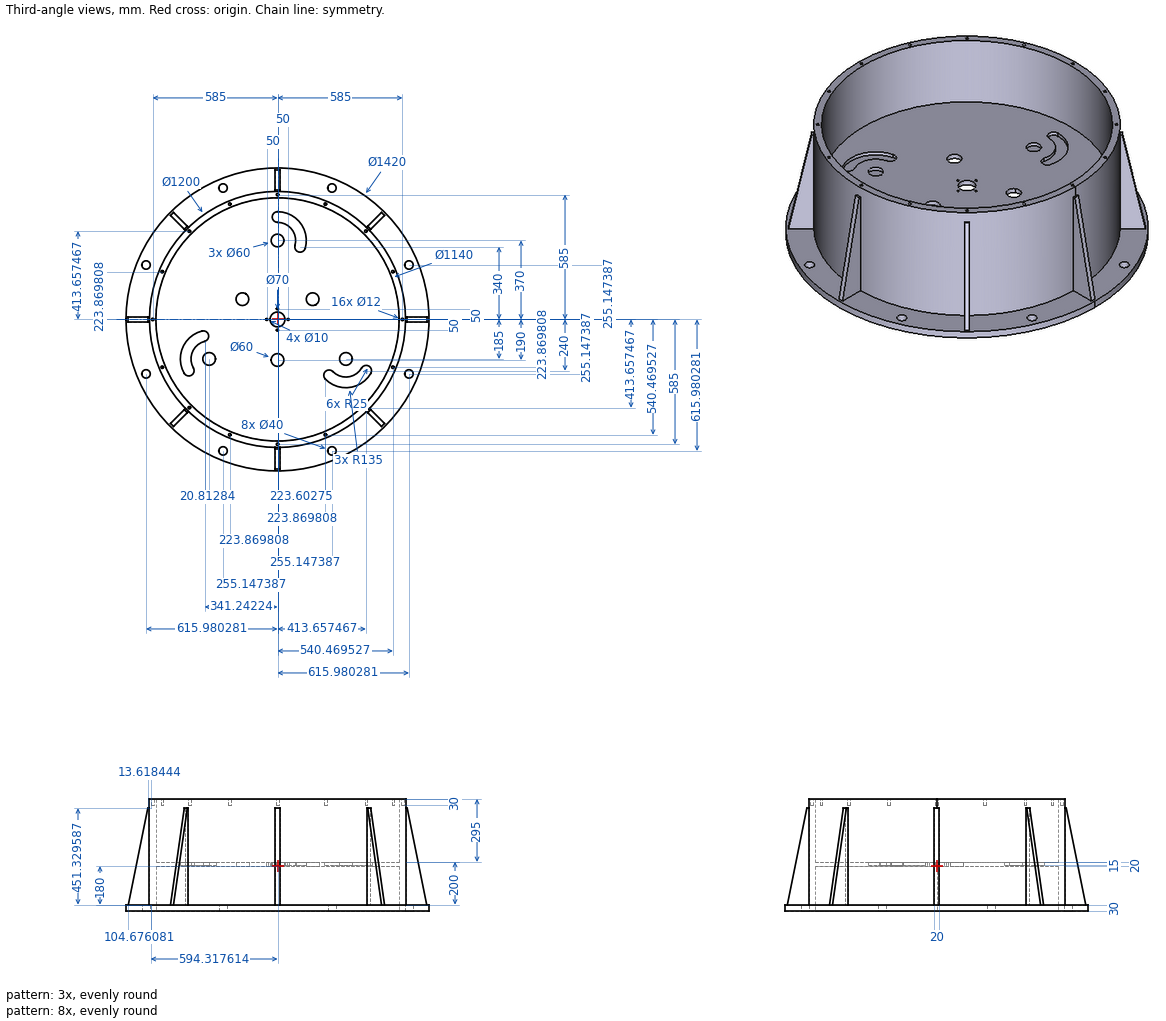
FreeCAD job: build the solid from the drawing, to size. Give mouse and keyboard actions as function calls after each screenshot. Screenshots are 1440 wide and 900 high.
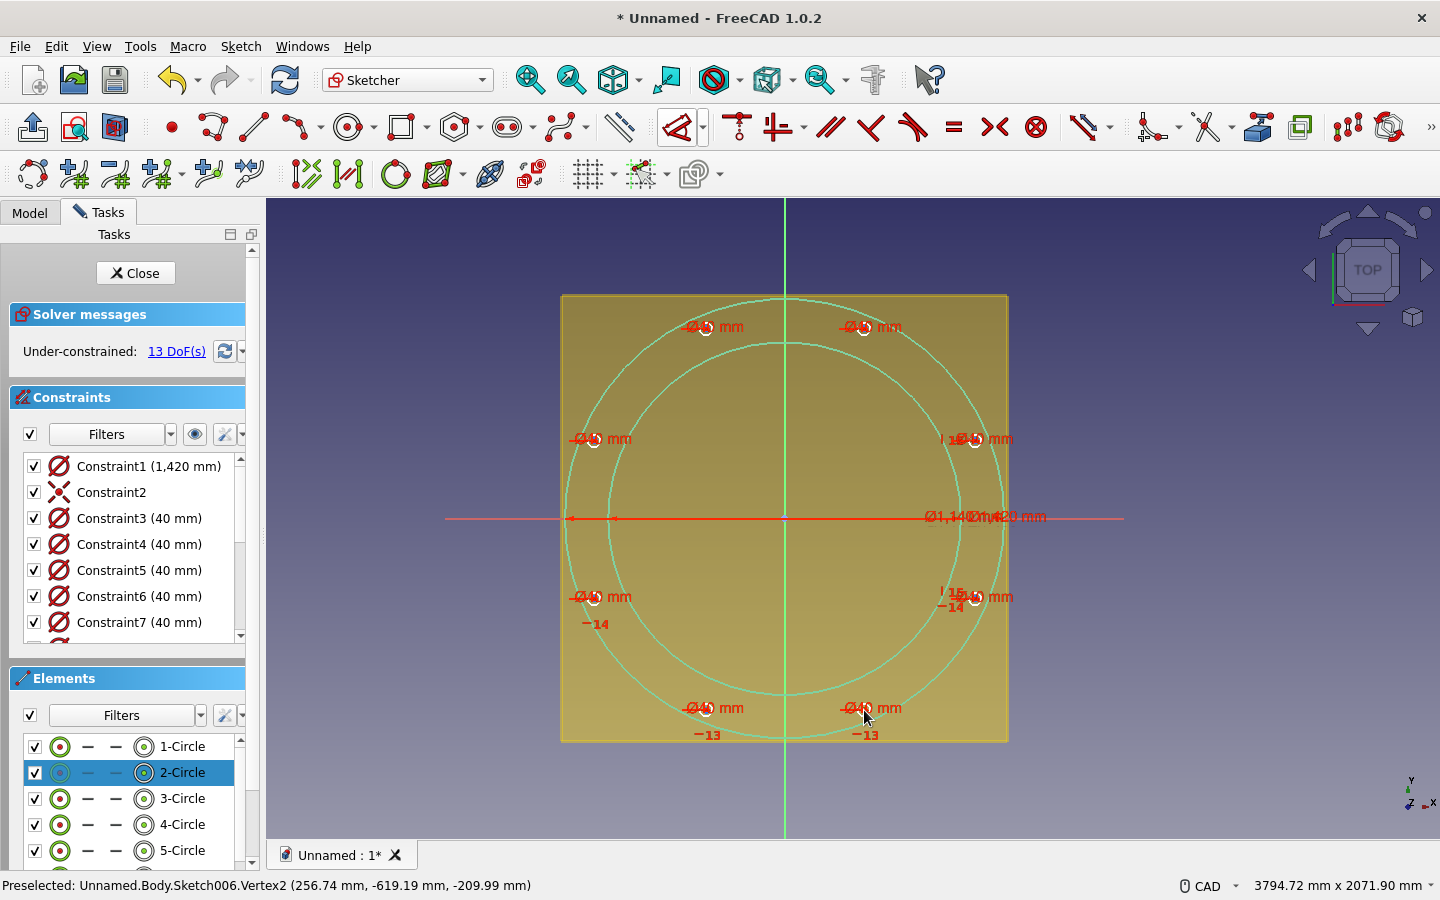
click(864, 329)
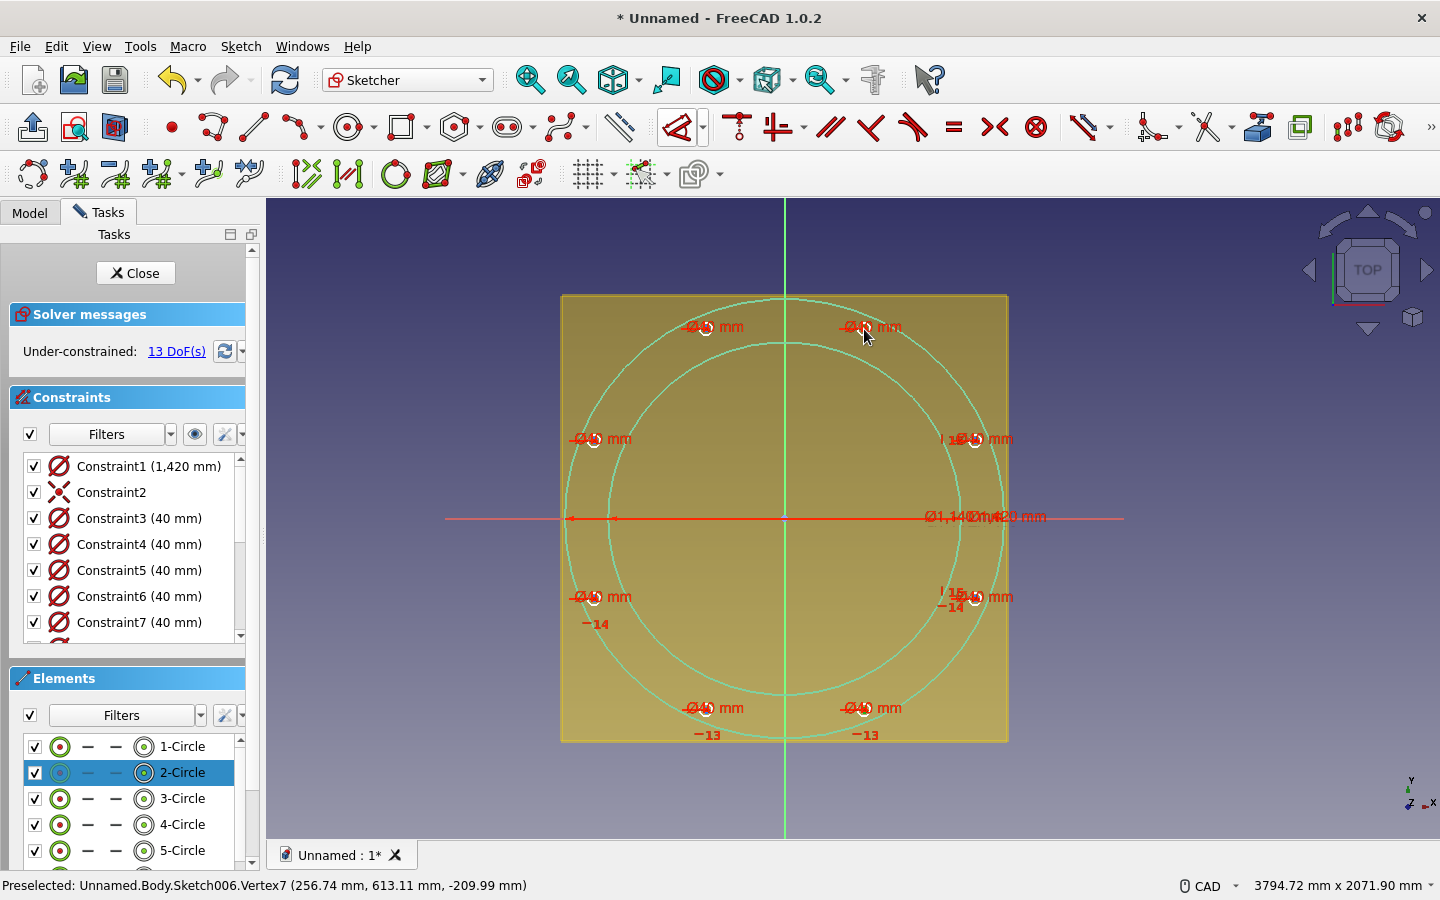
key(v)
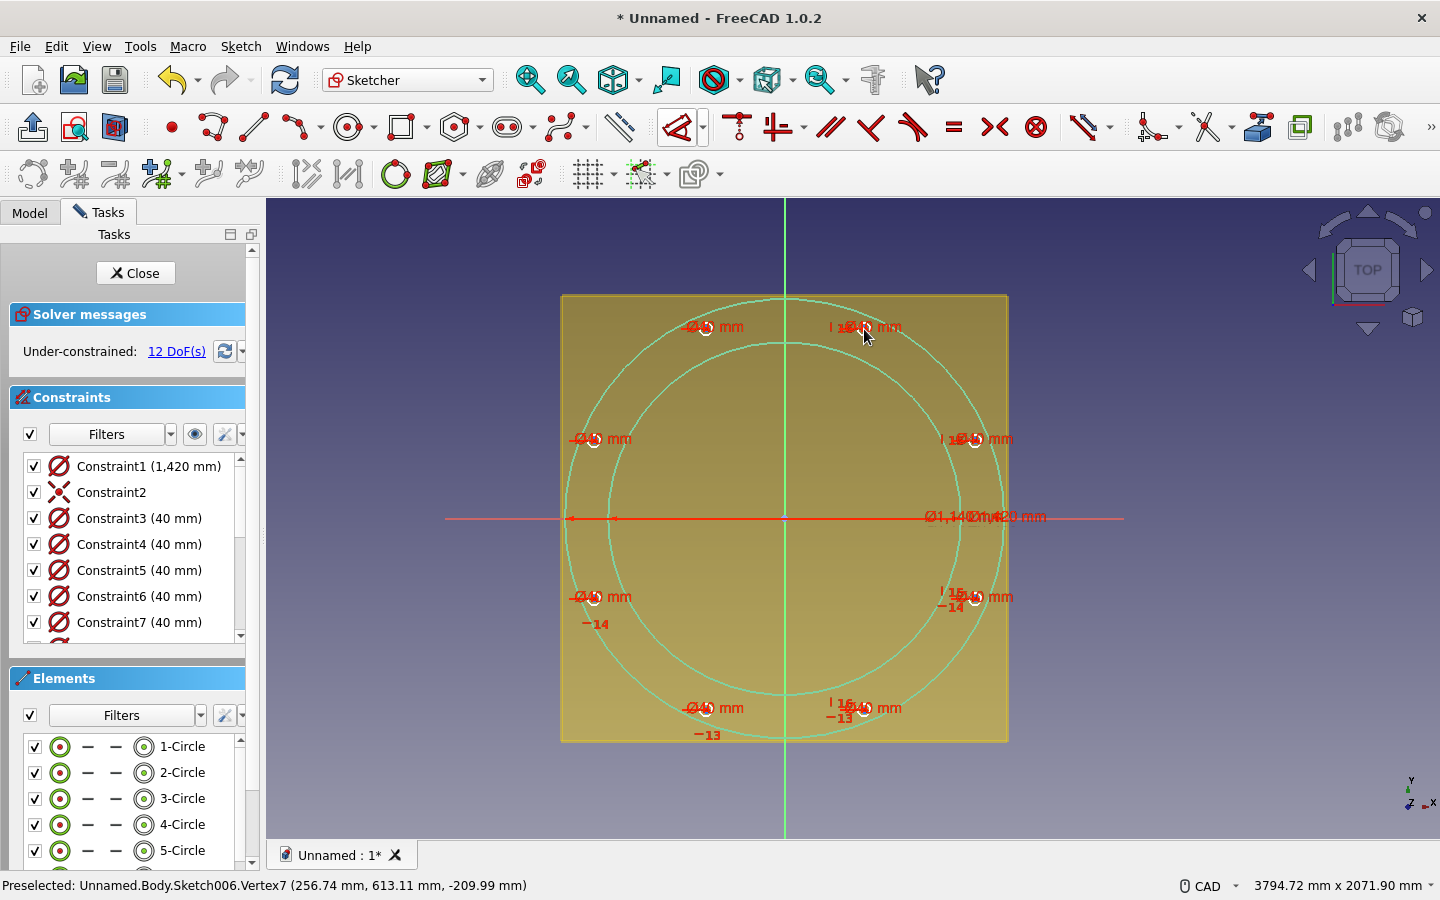
click(594, 599)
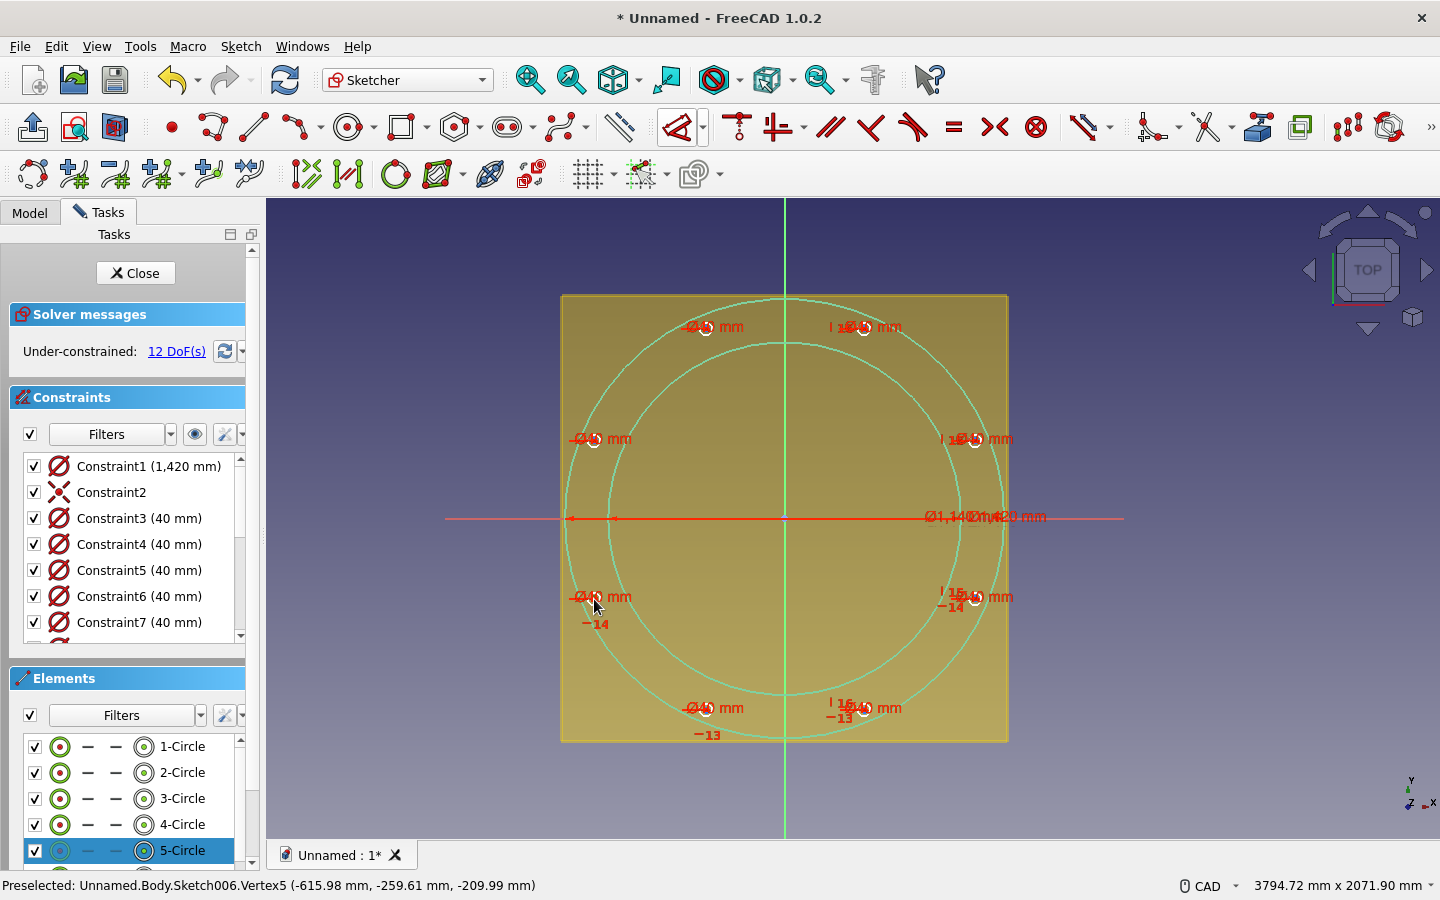
click(594, 441)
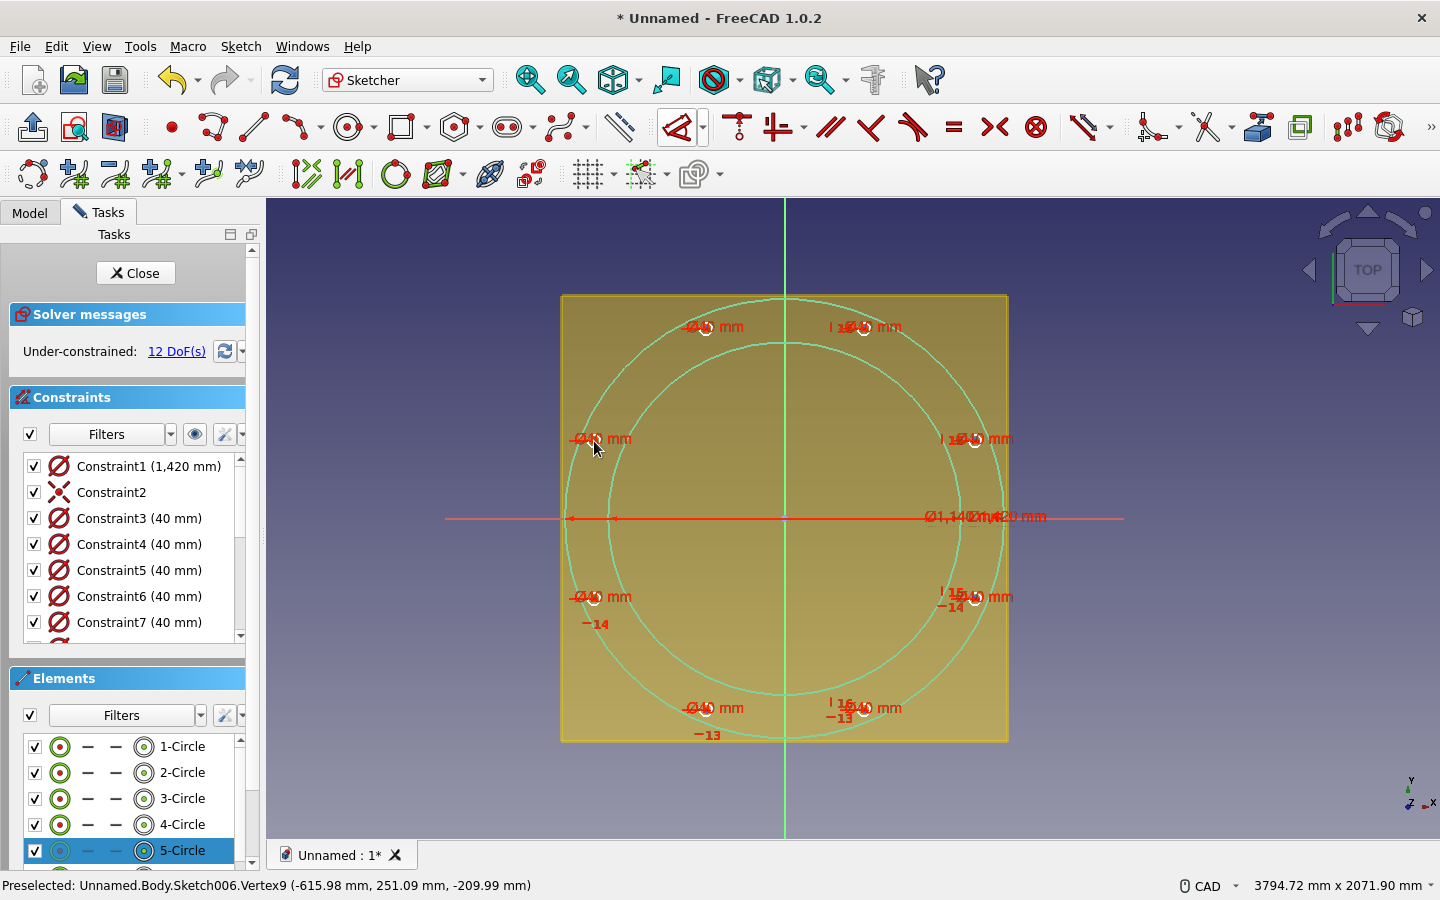
click(804, 128)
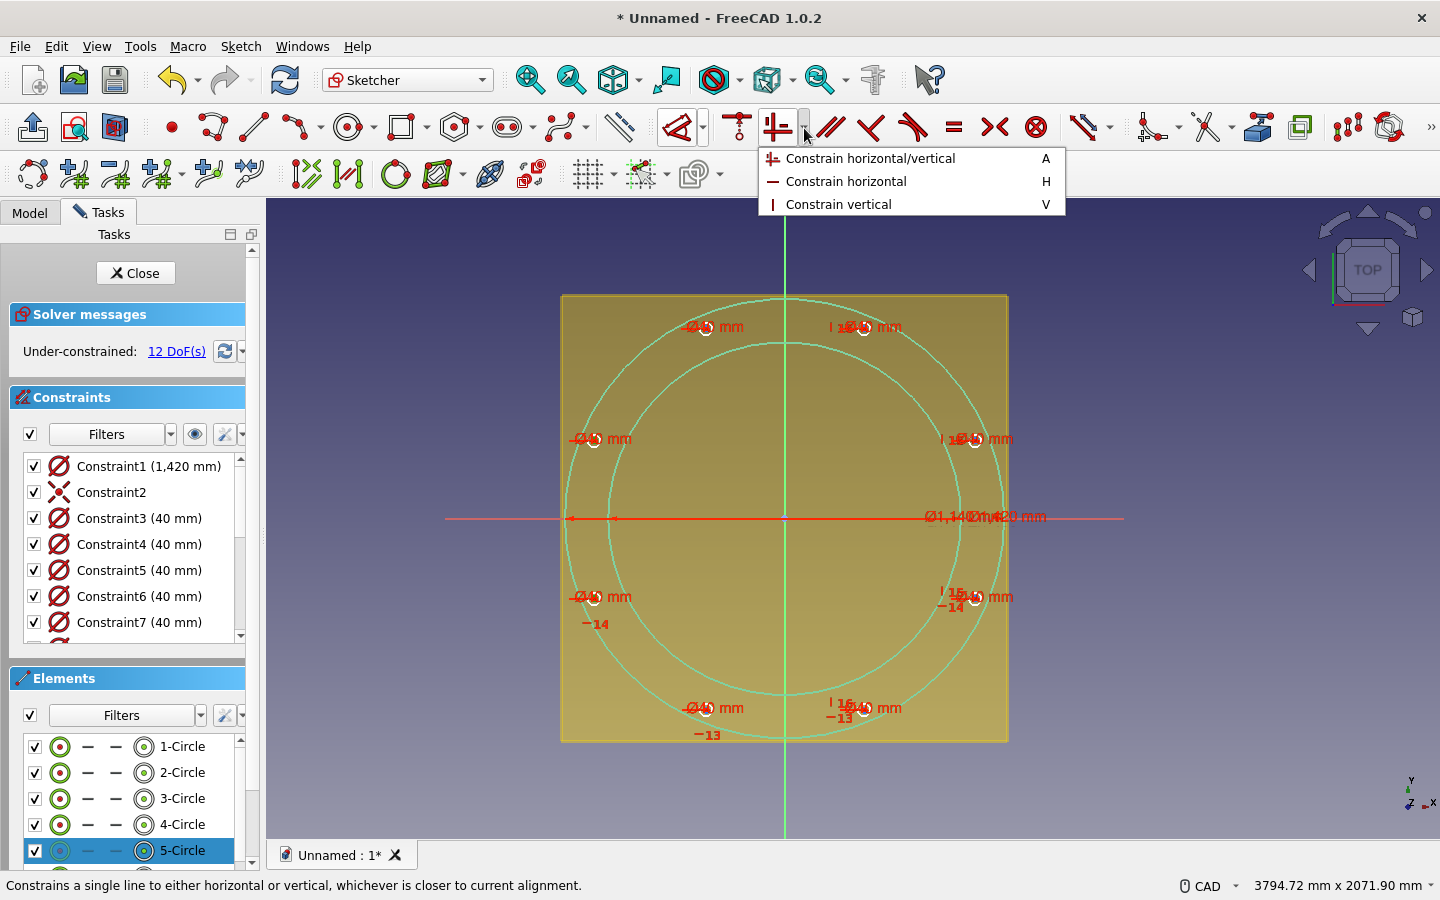
click(912, 204)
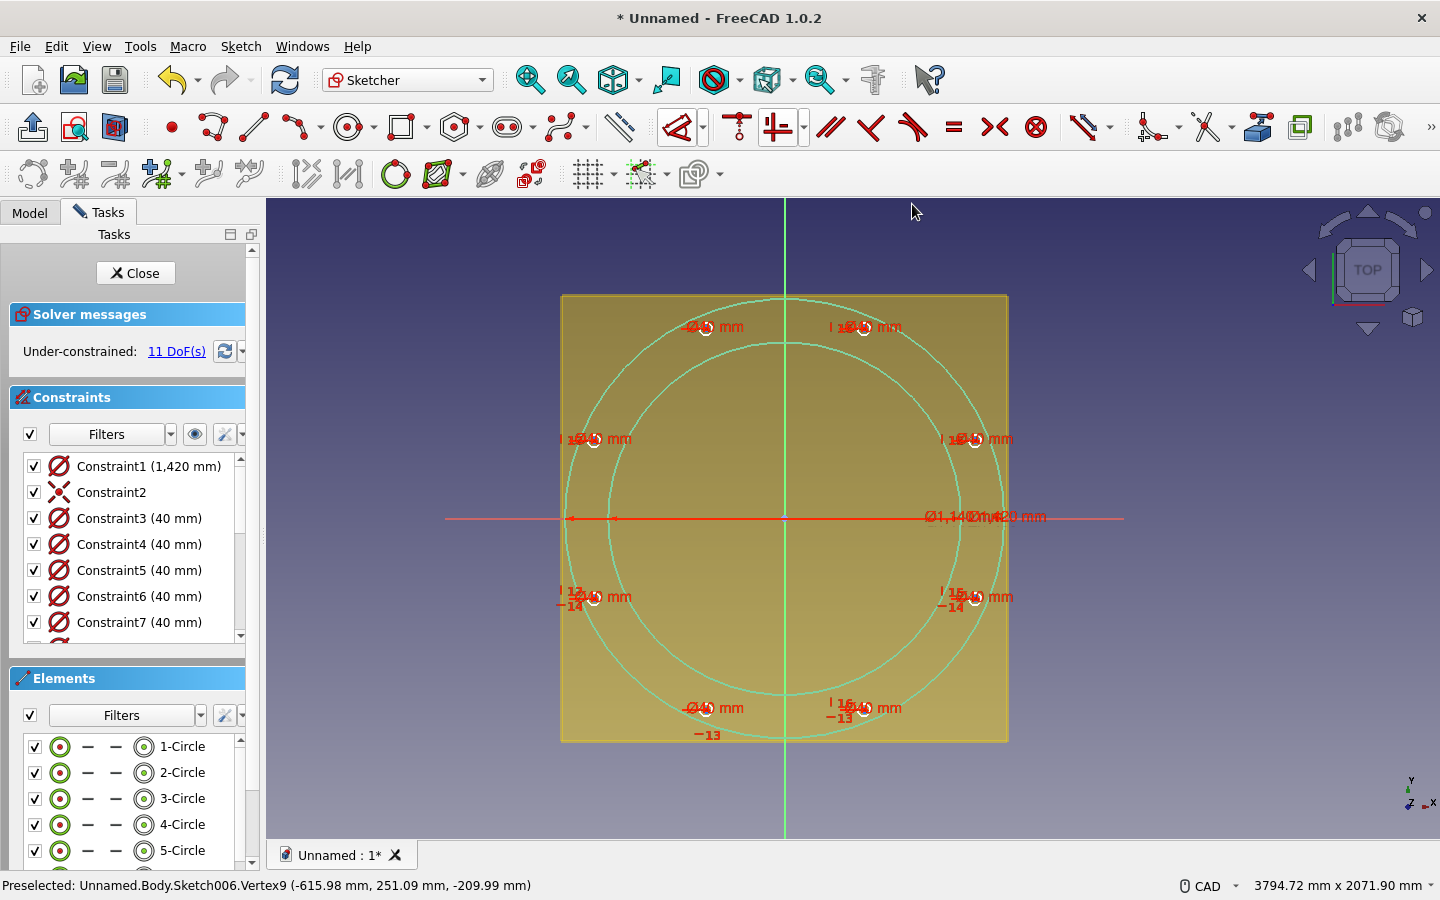
click(975, 441)